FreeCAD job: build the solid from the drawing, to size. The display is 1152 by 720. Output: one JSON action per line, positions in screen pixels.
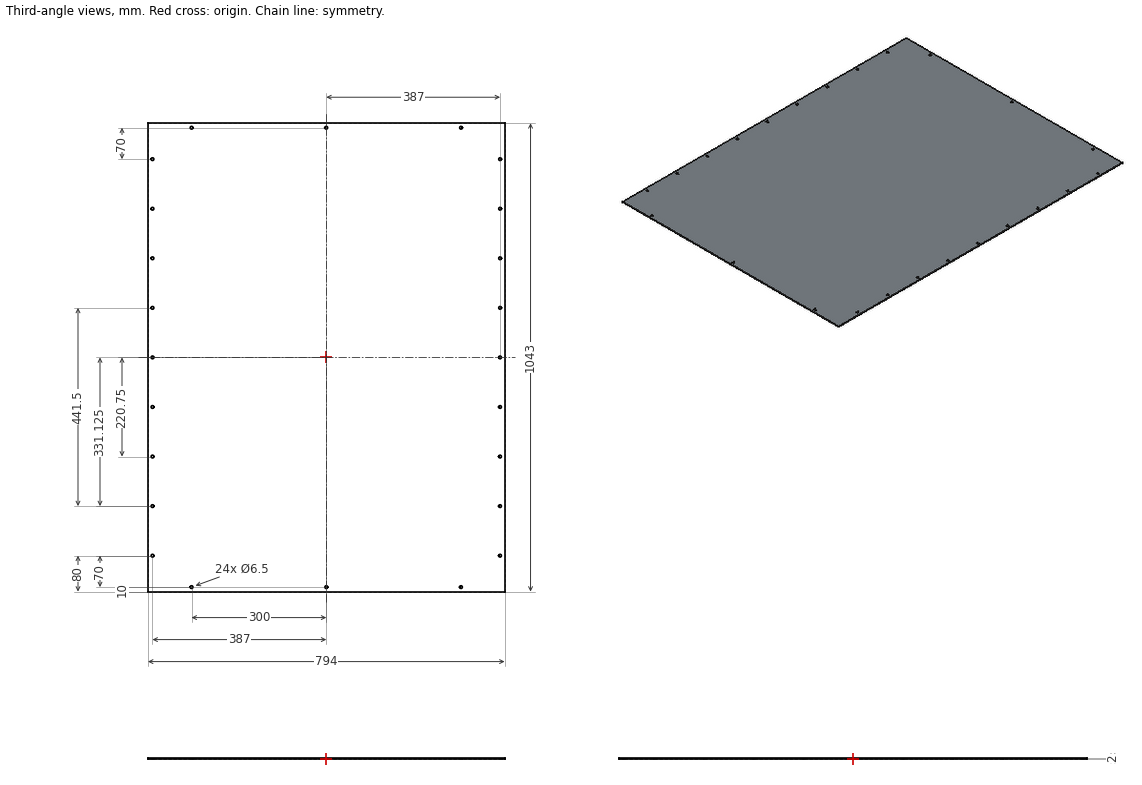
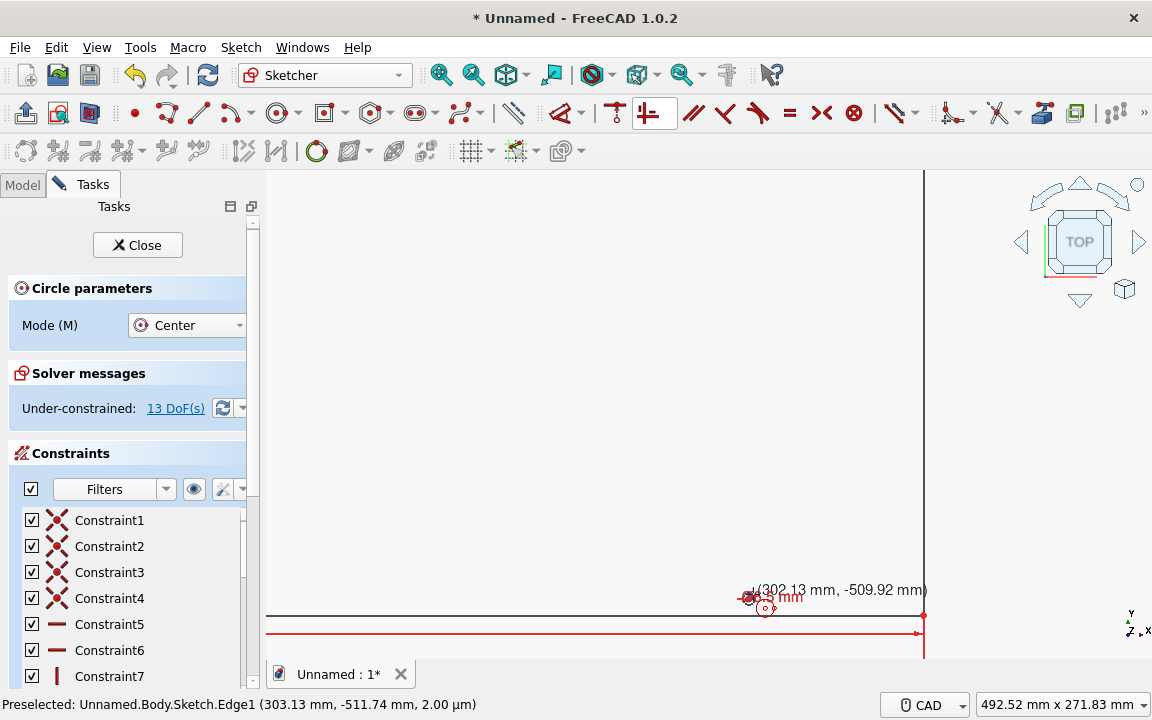
{"action": "scroll", "coordinate": [906, 472], "scroll_direction": "up", "scroll_amount": 7}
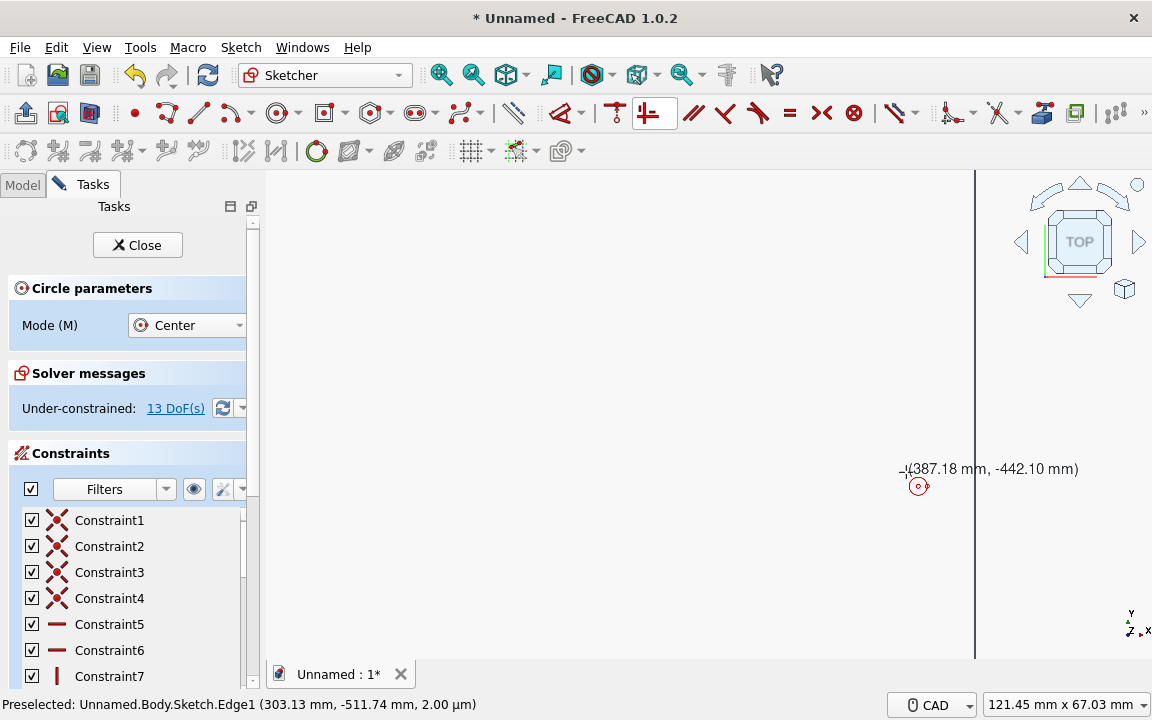
{"action": "scroll", "coordinate": [775, 580], "scroll_direction": "down", "scroll_amount": 15}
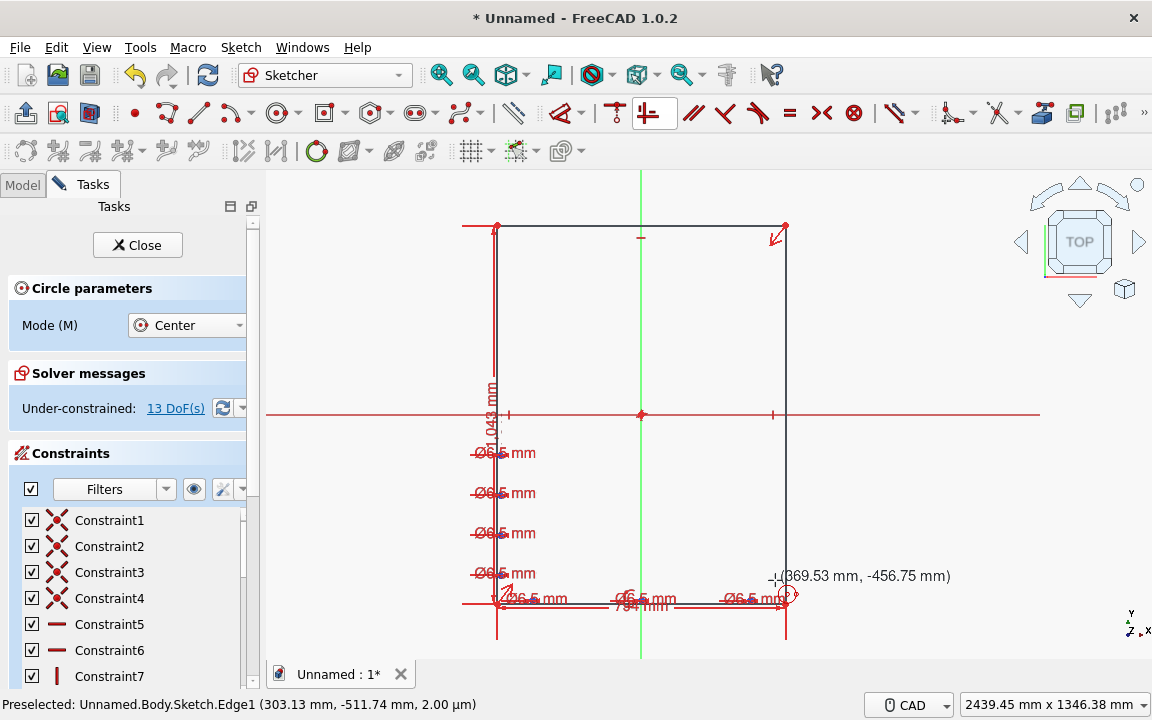
{"action": "scroll", "coordinate": [782, 575], "scroll_direction": "up", "scroll_amount": 8}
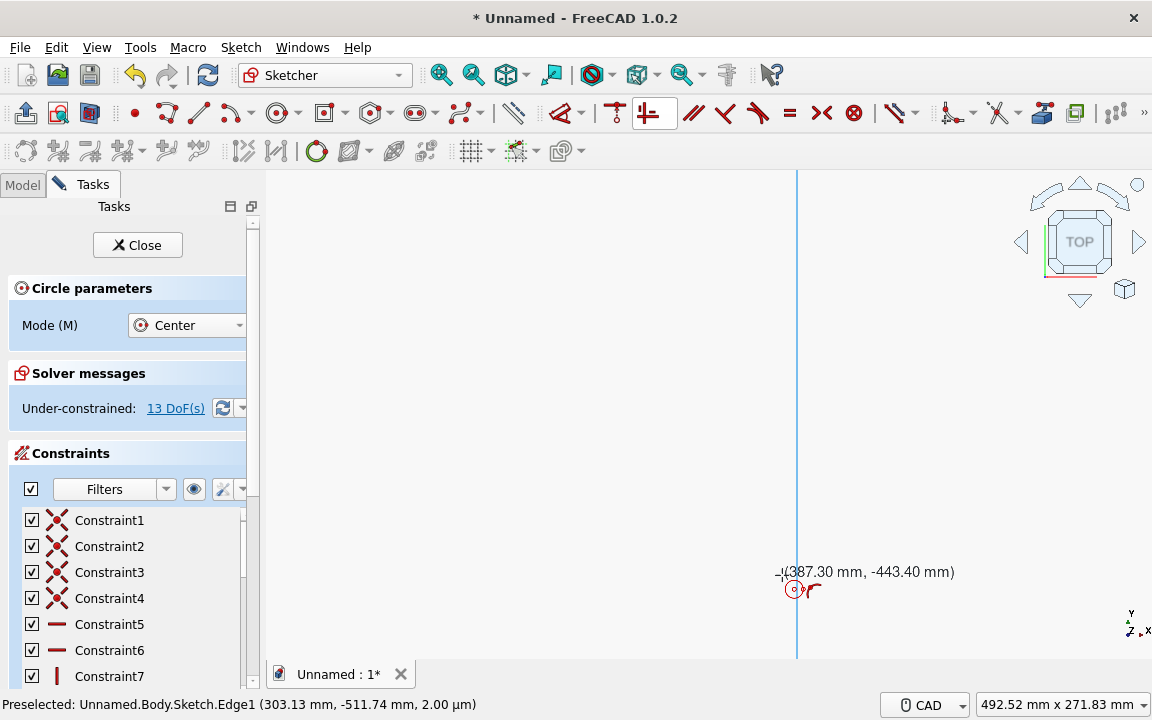
{"action": "left_click", "coordinate": [779, 573]}
{"action": "mouse_move", "coordinate": [775, 569]}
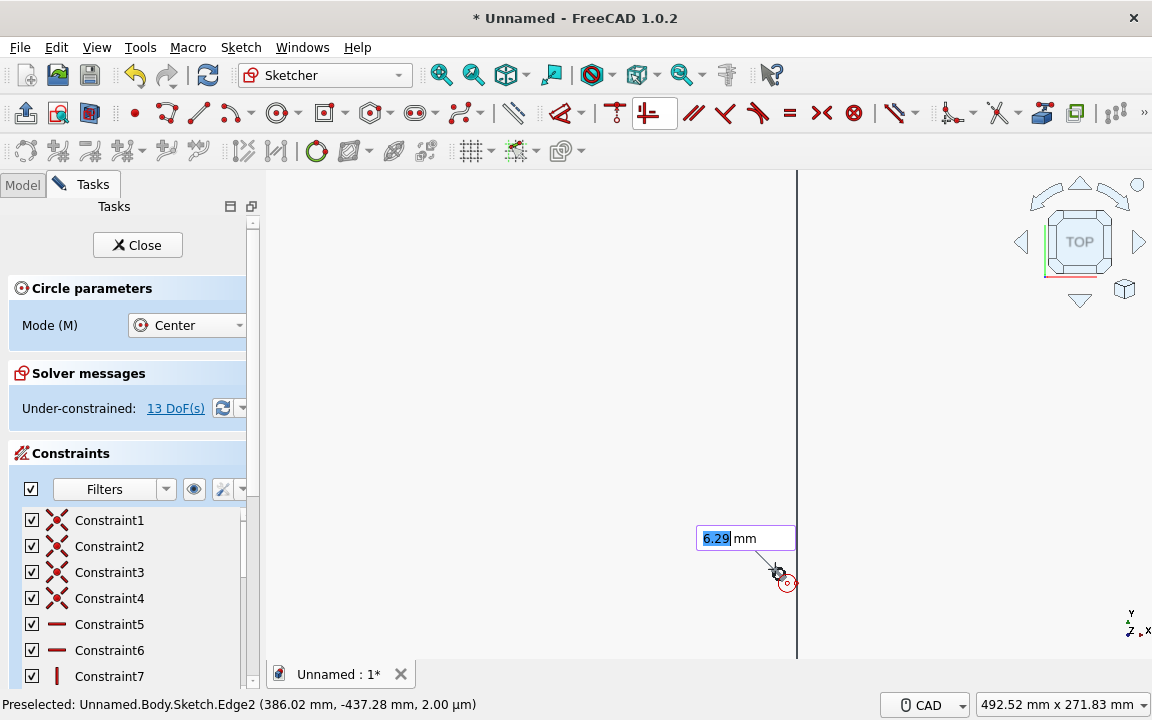
{"action": "type", "text": "6.5"}
{"action": "key", "text": "Return"}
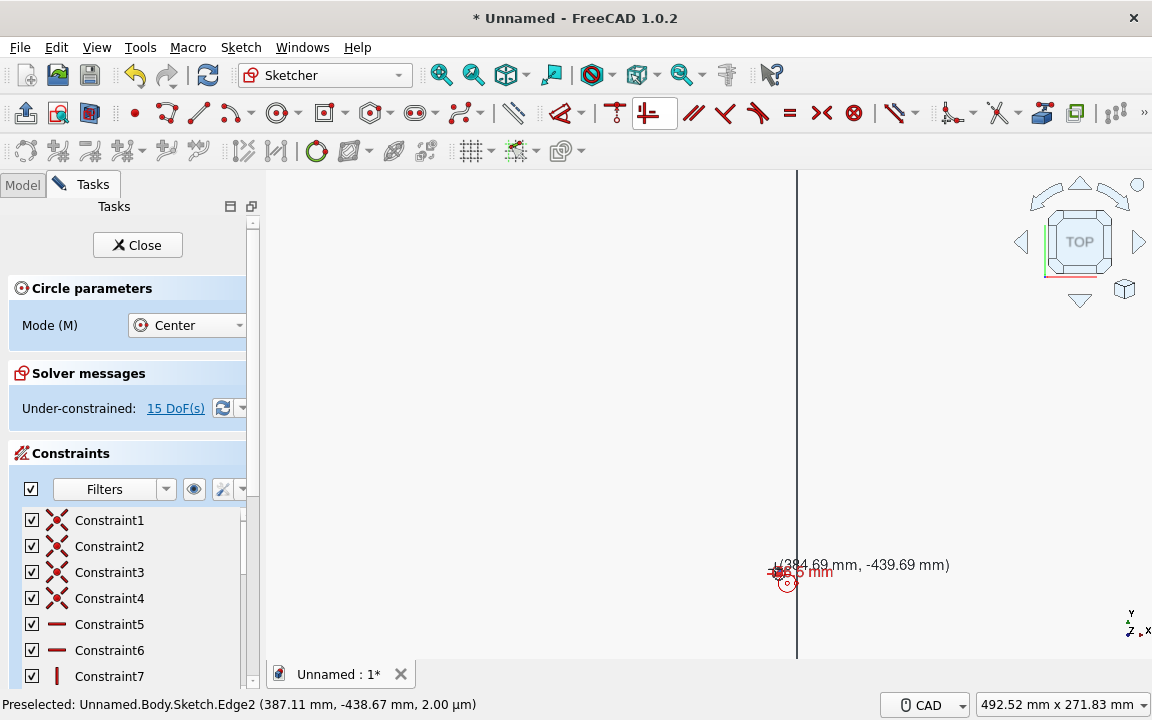
{"action": "scroll", "coordinate": [779, 375], "scroll_direction": "up", "scroll_amount": 7}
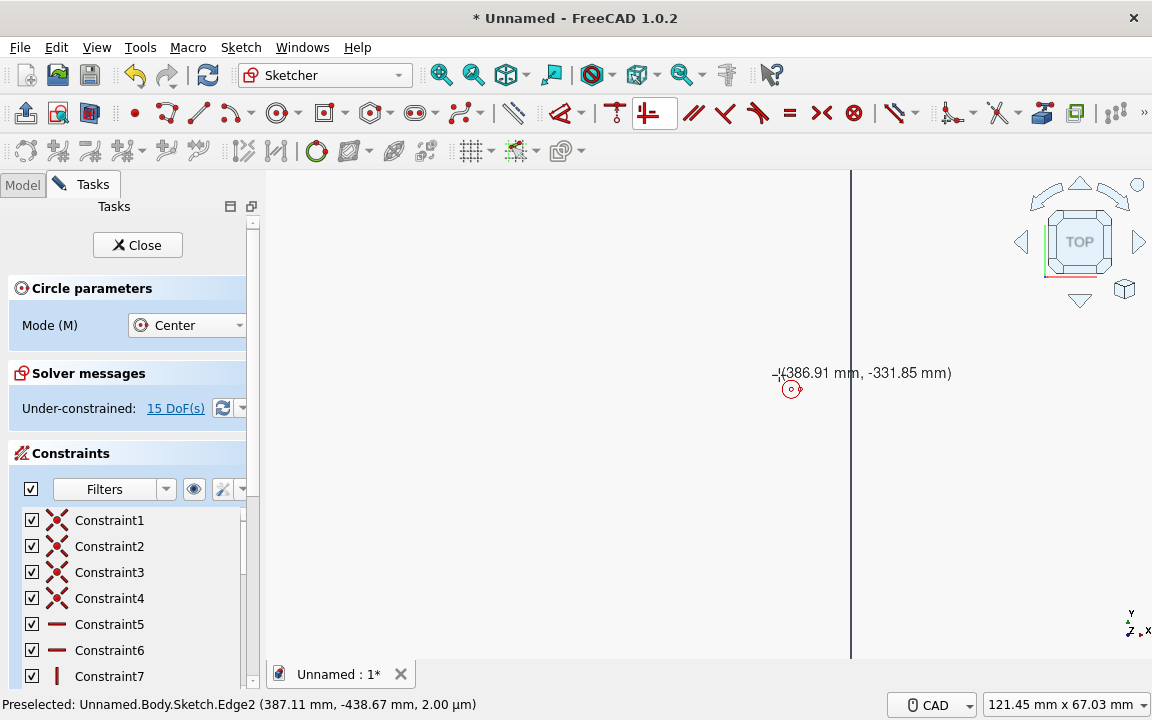
{"action": "scroll", "coordinate": [781, 543], "scroll_direction": "down", "scroll_amount": 15}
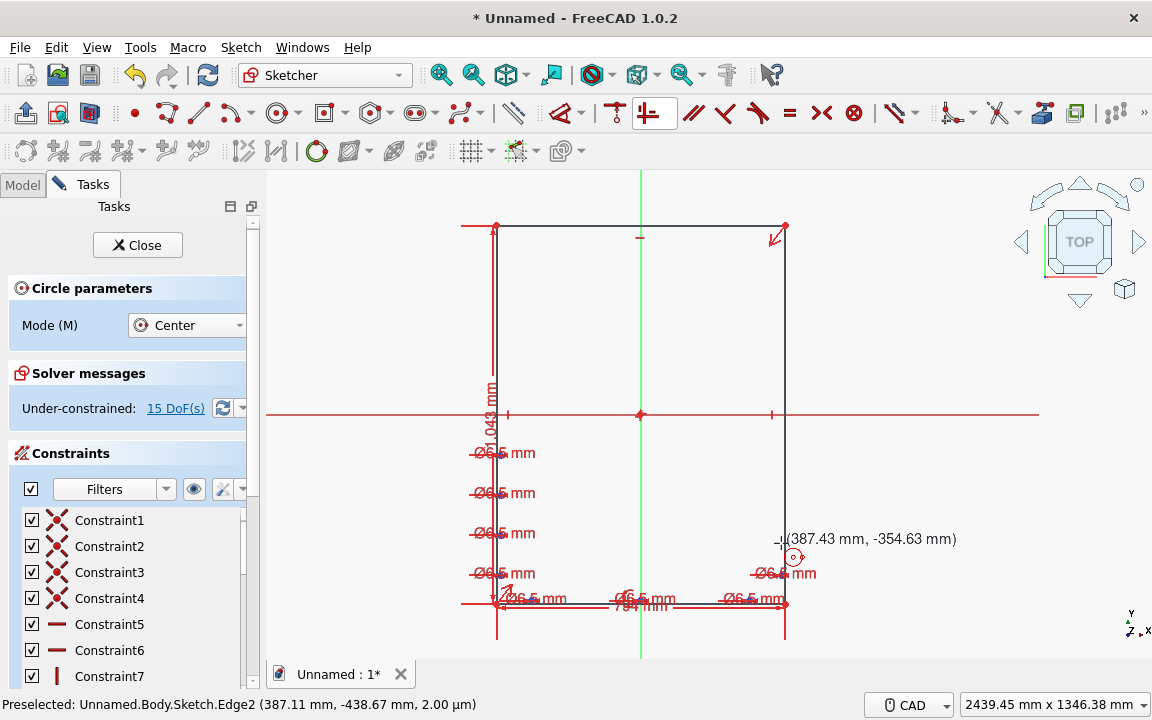
{"action": "scroll", "coordinate": [781, 535], "scroll_direction": "up", "scroll_amount": 8}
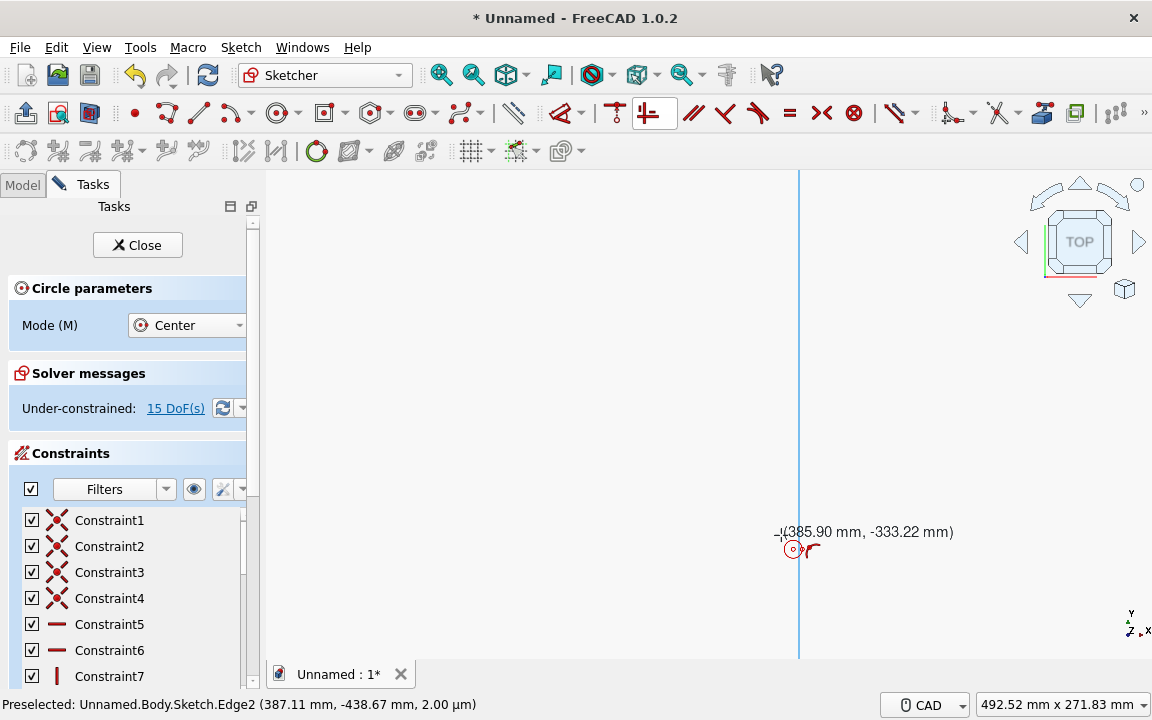
{"action": "left_click", "coordinate": [781, 533]}
{"action": "mouse_move", "coordinate": [777, 529]}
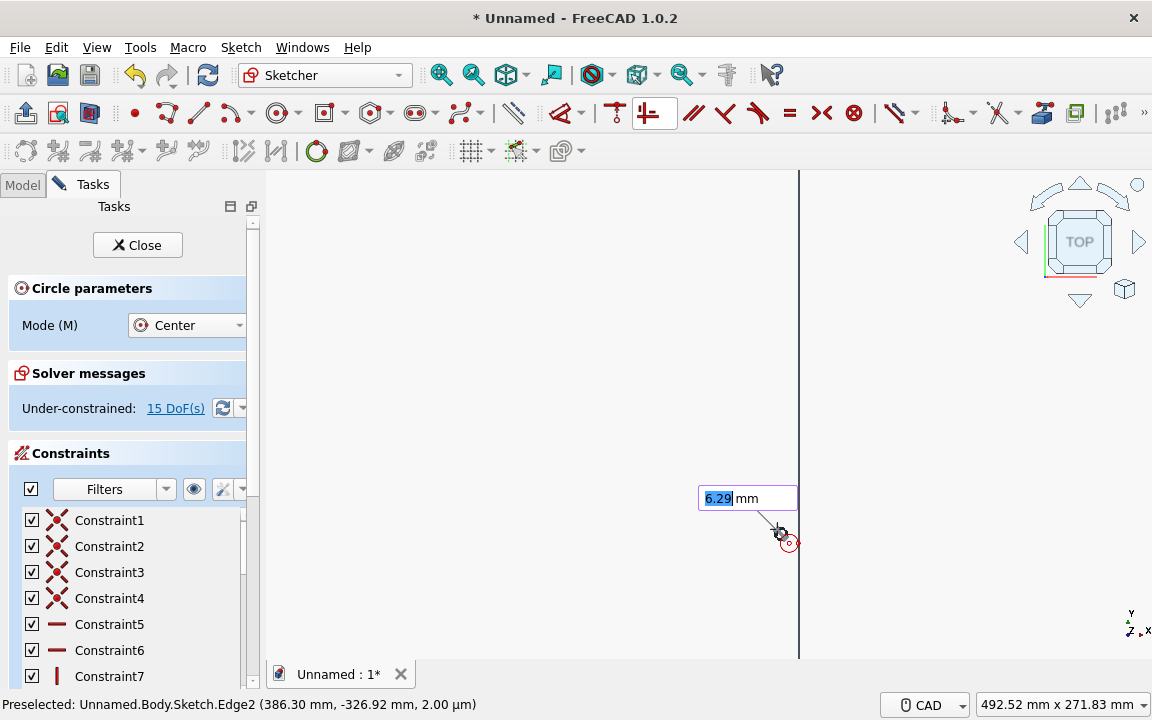
{"action": "type", "text": "6.5"}
{"action": "key", "text": "Return"}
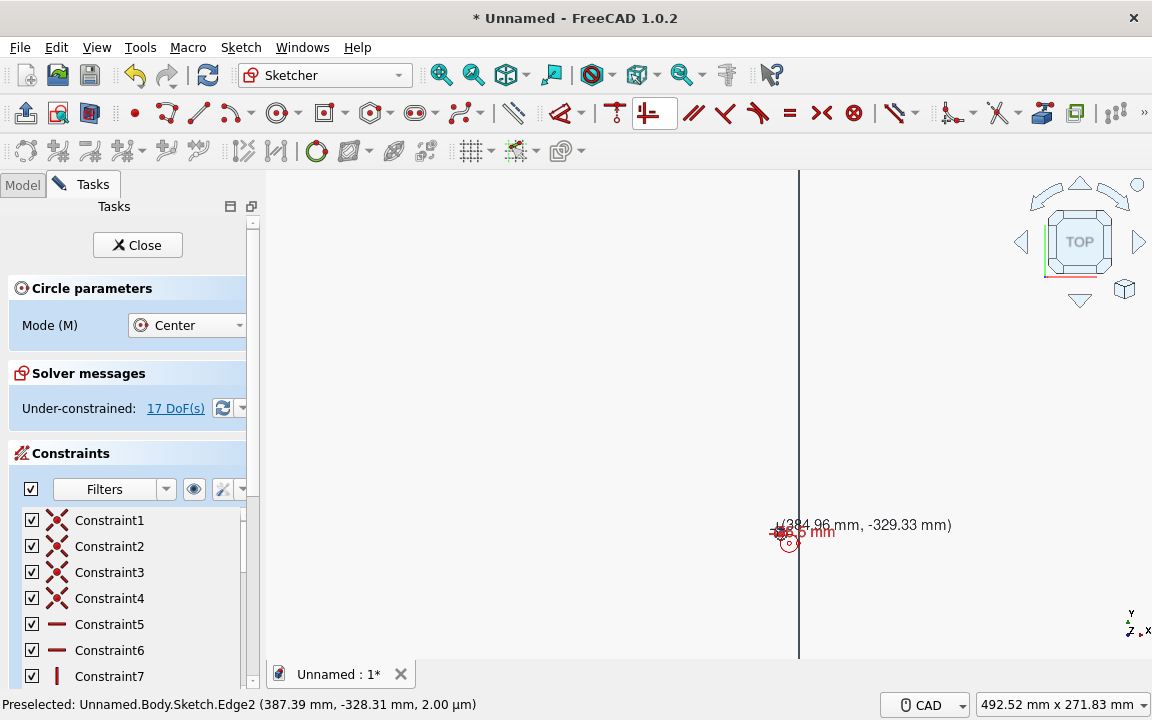
{"action": "scroll", "coordinate": [781, 335], "scroll_direction": "up", "scroll_amount": 7}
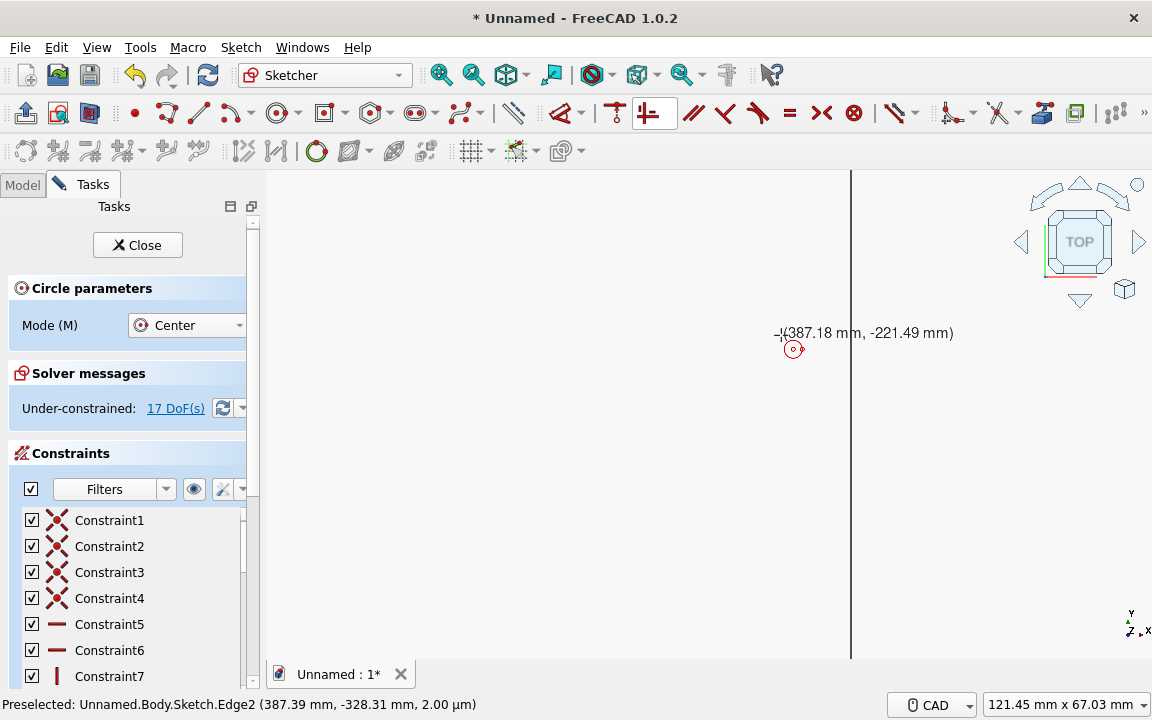
{"action": "scroll", "coordinate": [781, 503], "scroll_direction": "down", "scroll_amount": 15}